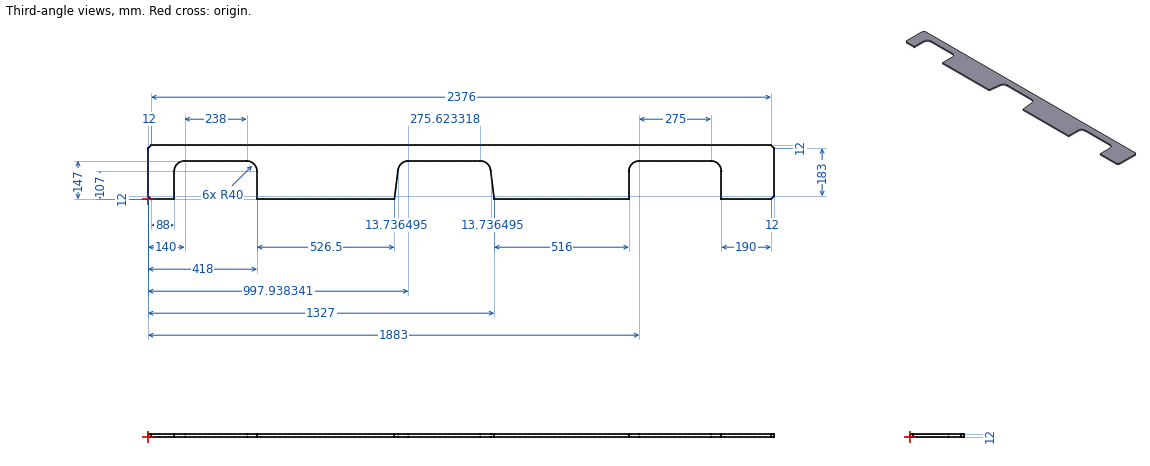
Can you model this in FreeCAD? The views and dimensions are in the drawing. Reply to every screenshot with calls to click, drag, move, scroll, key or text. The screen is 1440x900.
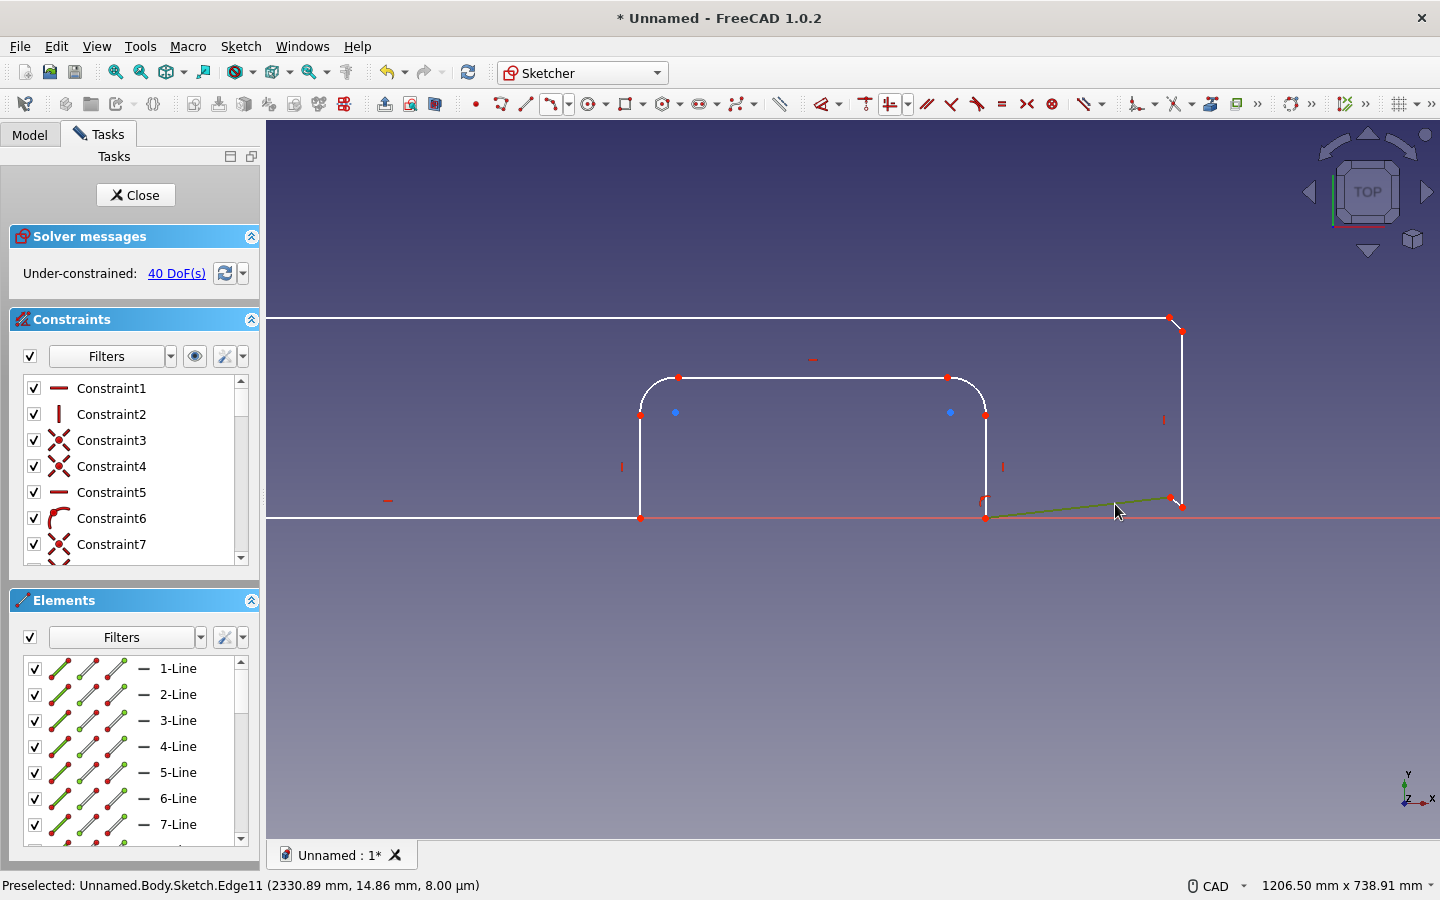
click(908, 104)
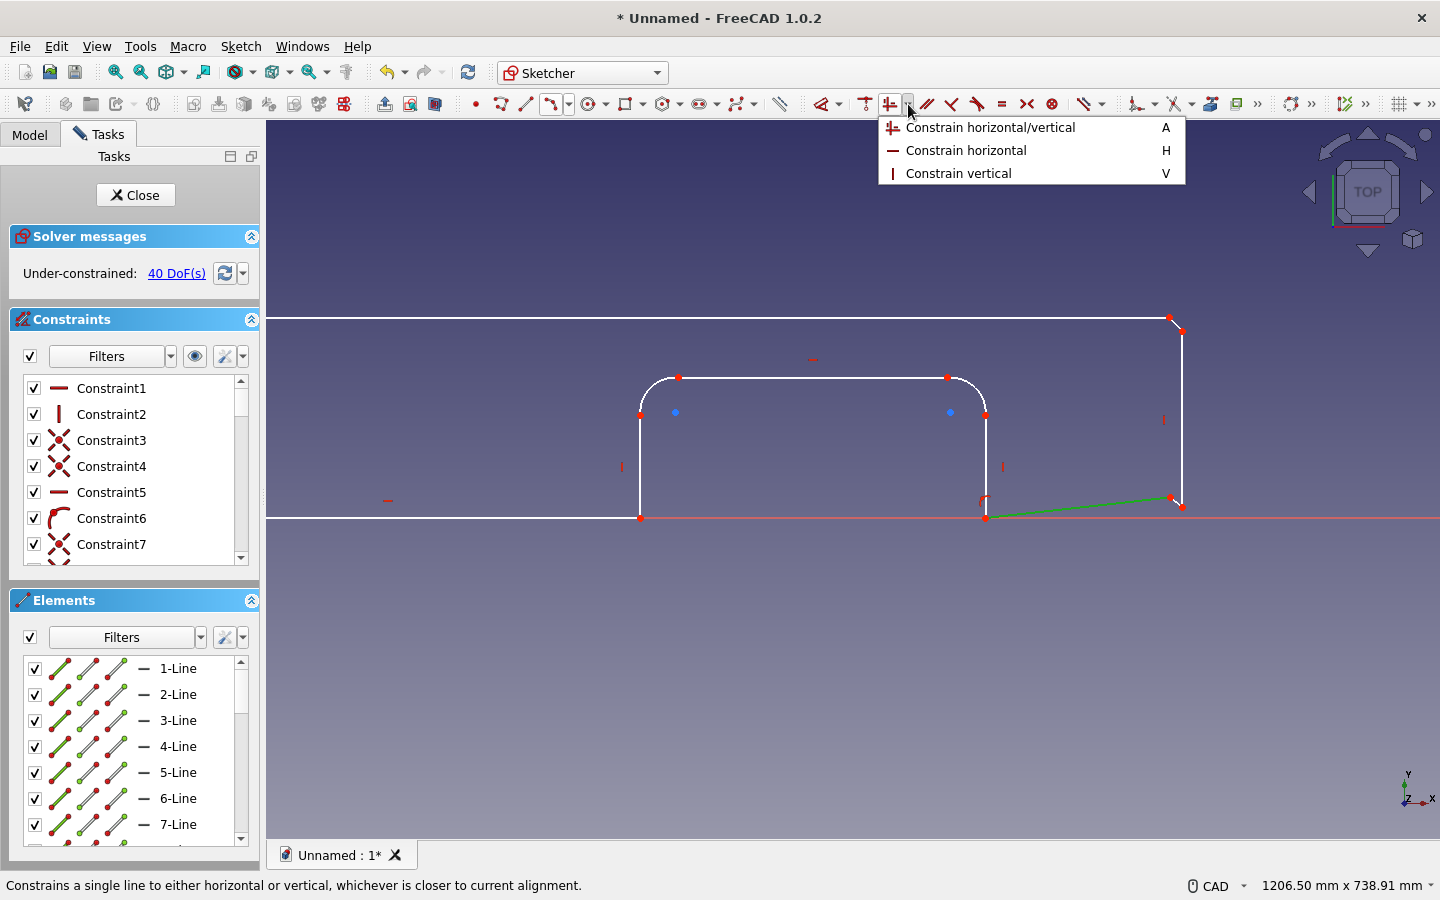
click(1032, 150)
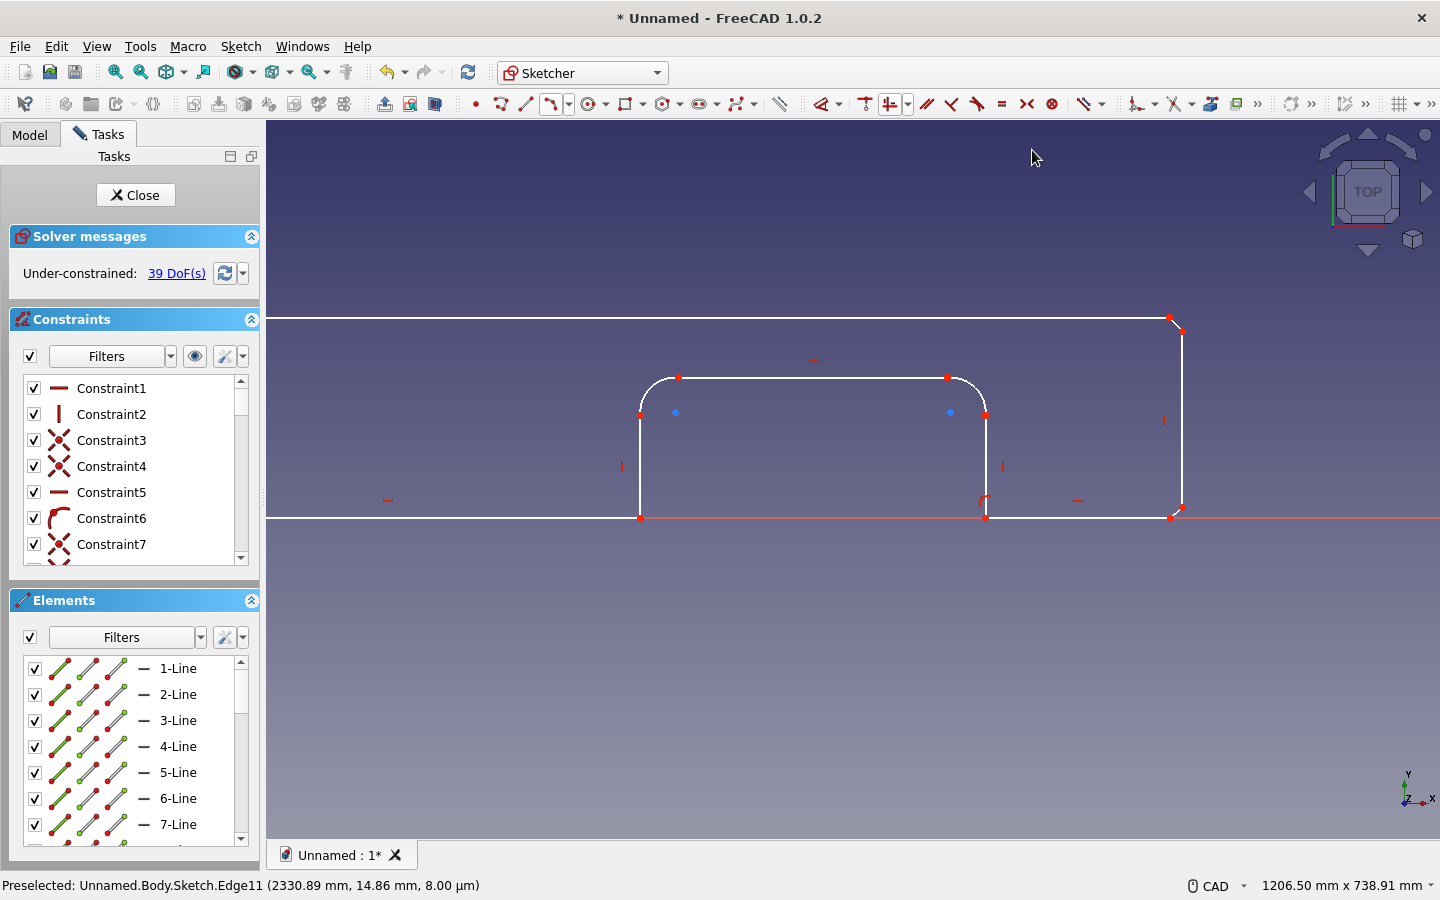
scroll(1116, 506, down, 6)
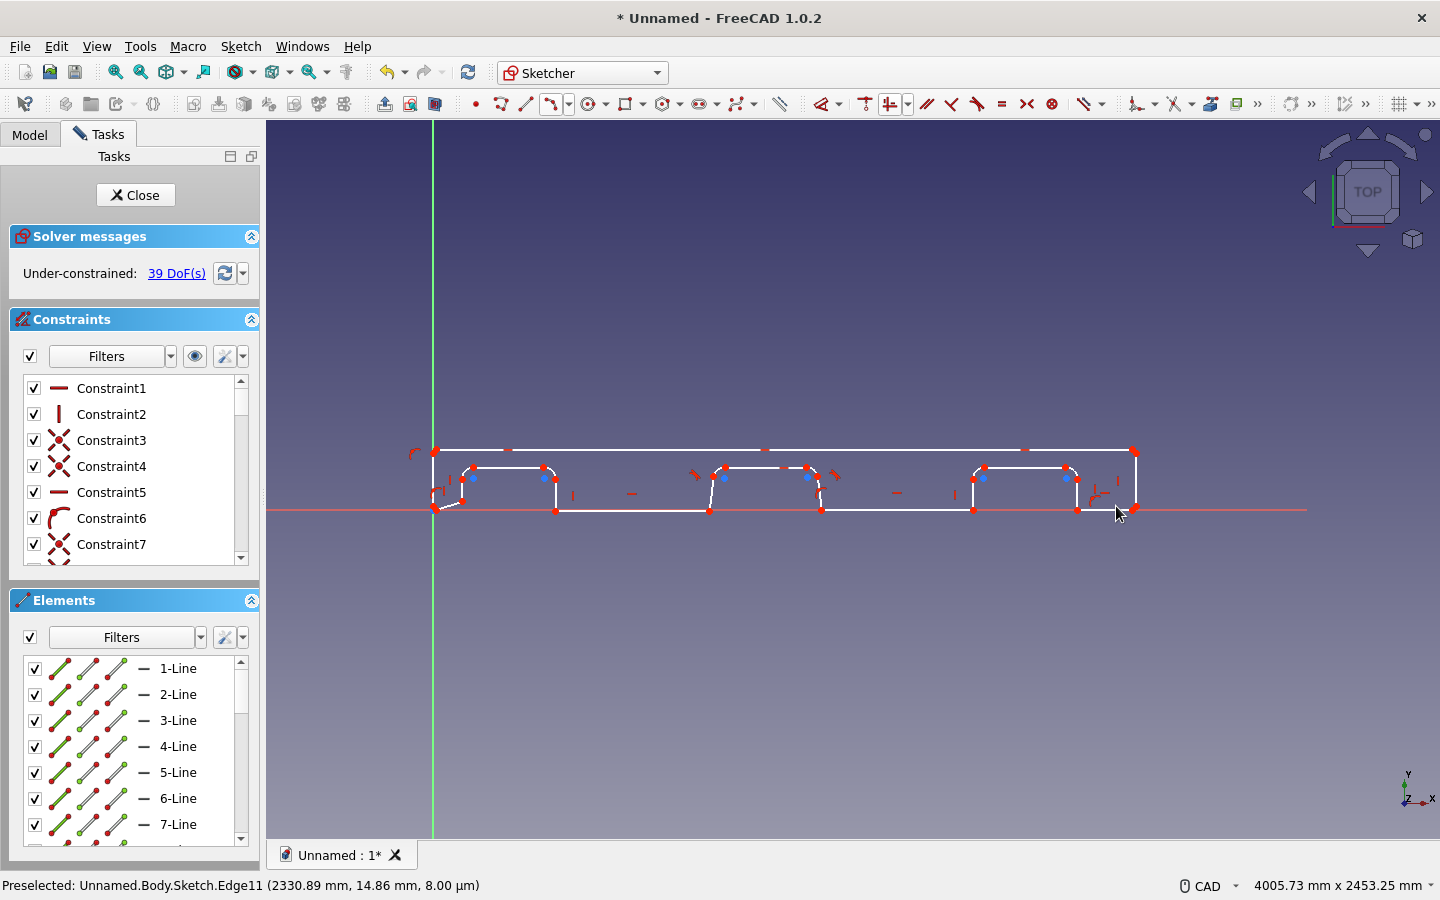
scroll(455, 504, up, 5)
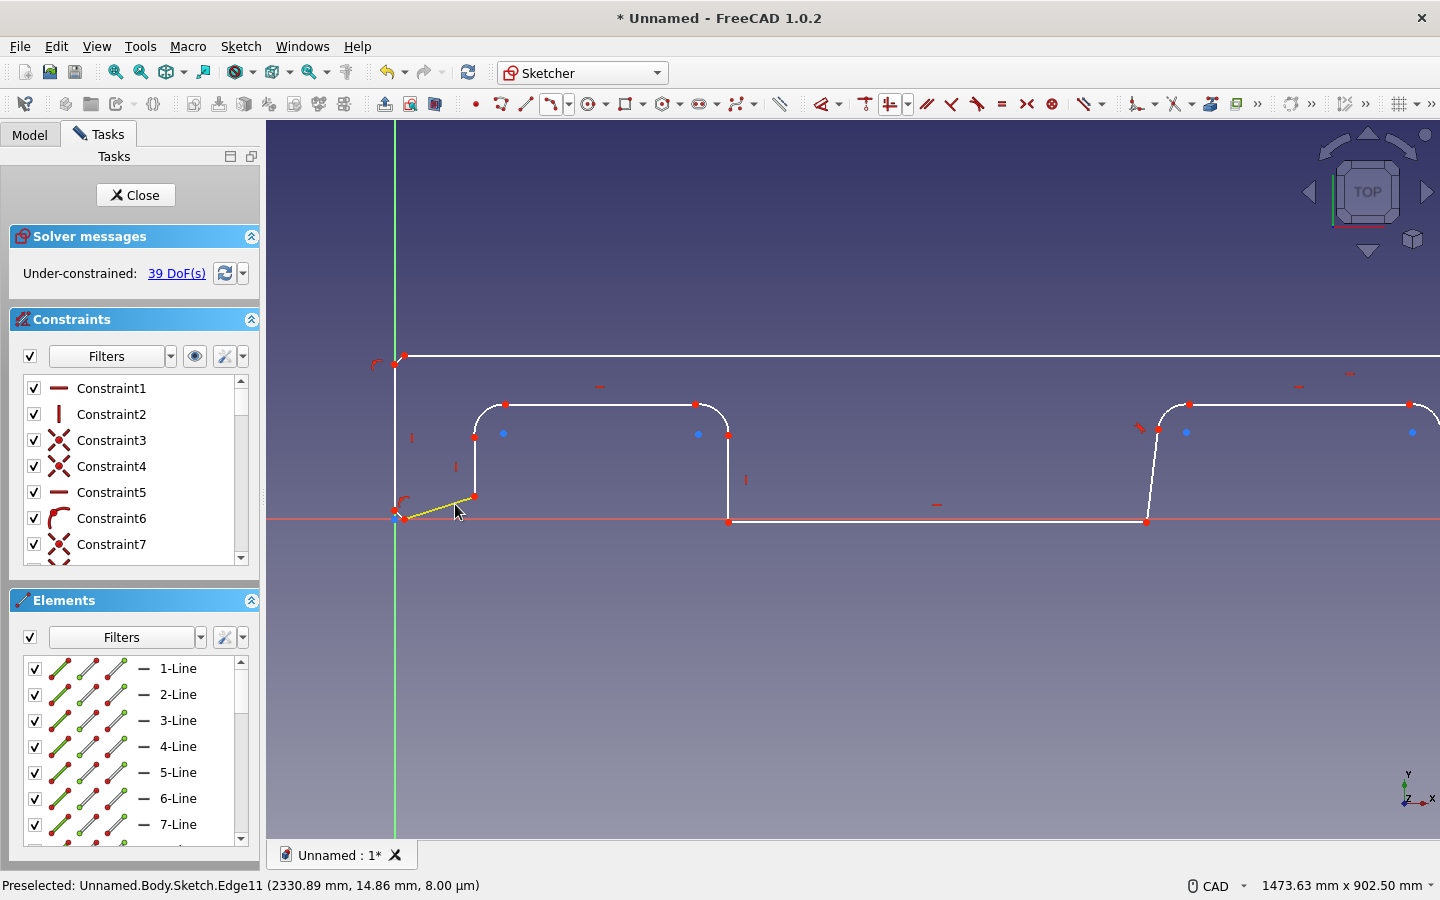
click(454, 504)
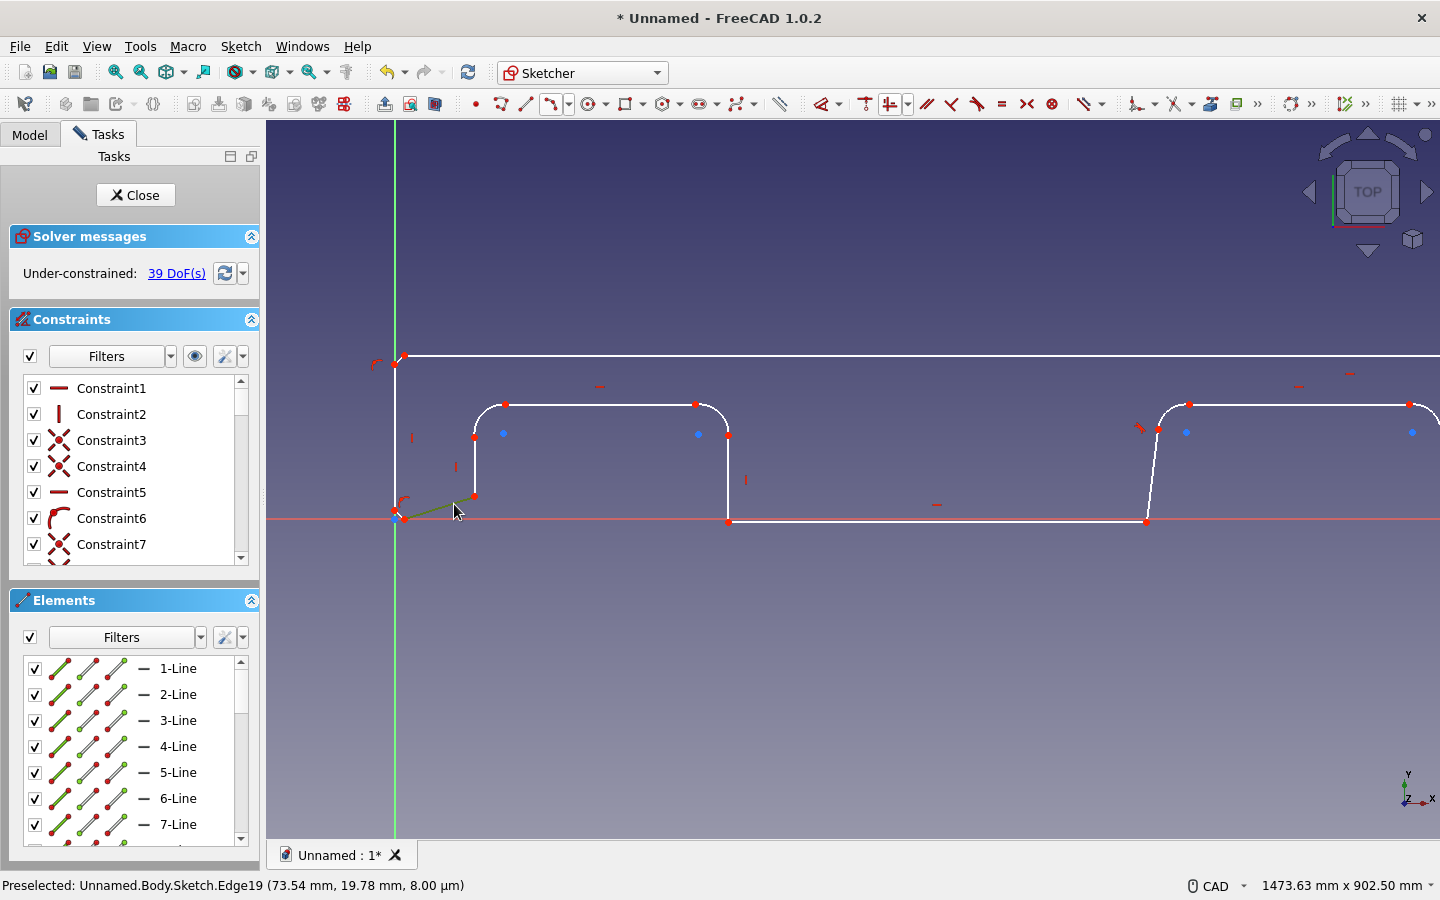
click(908, 104)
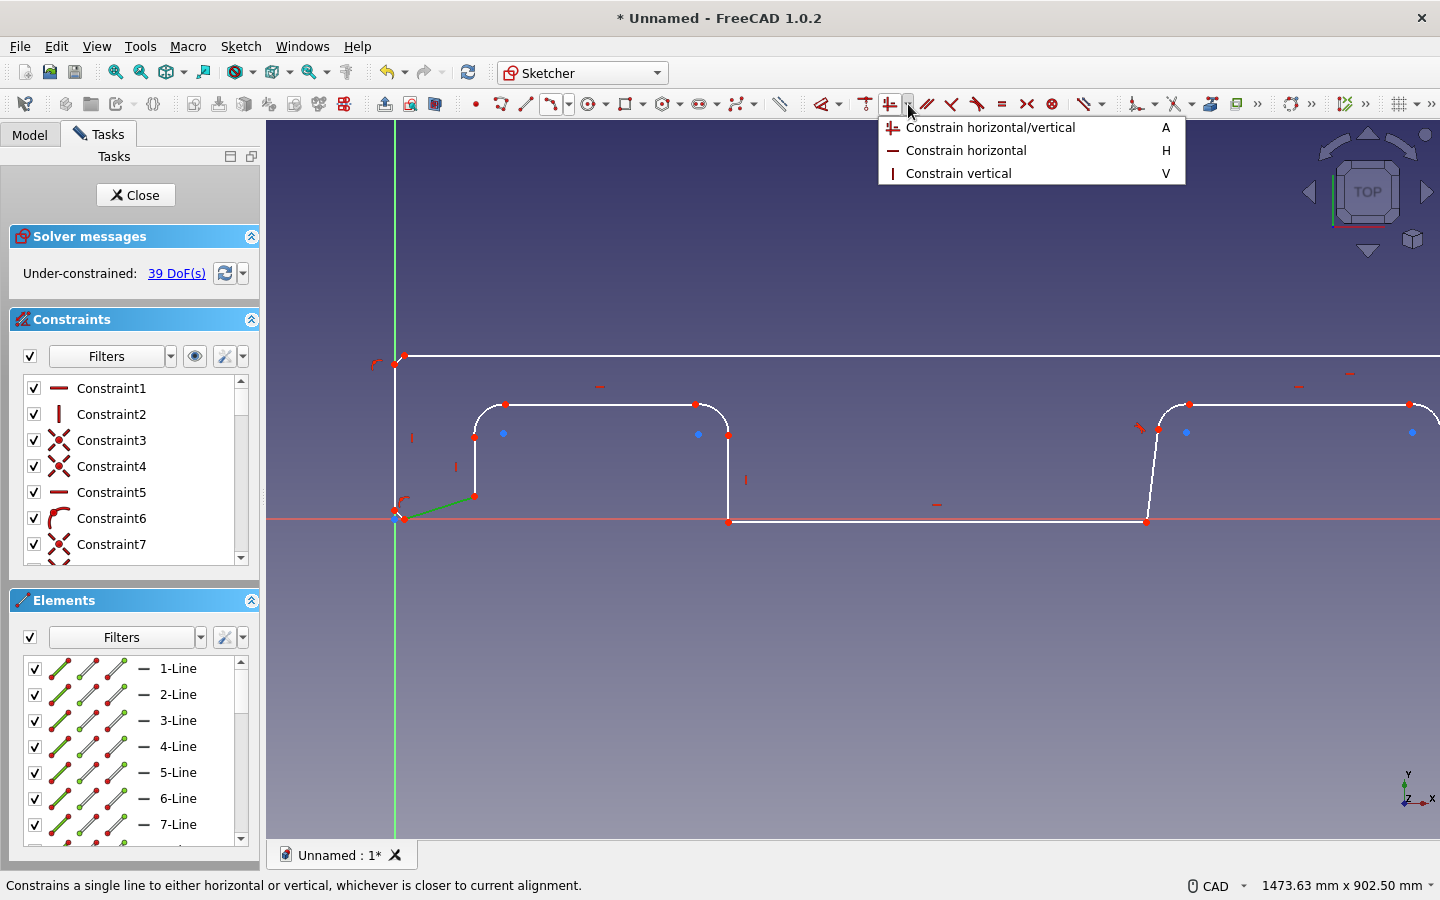
click(1032, 150)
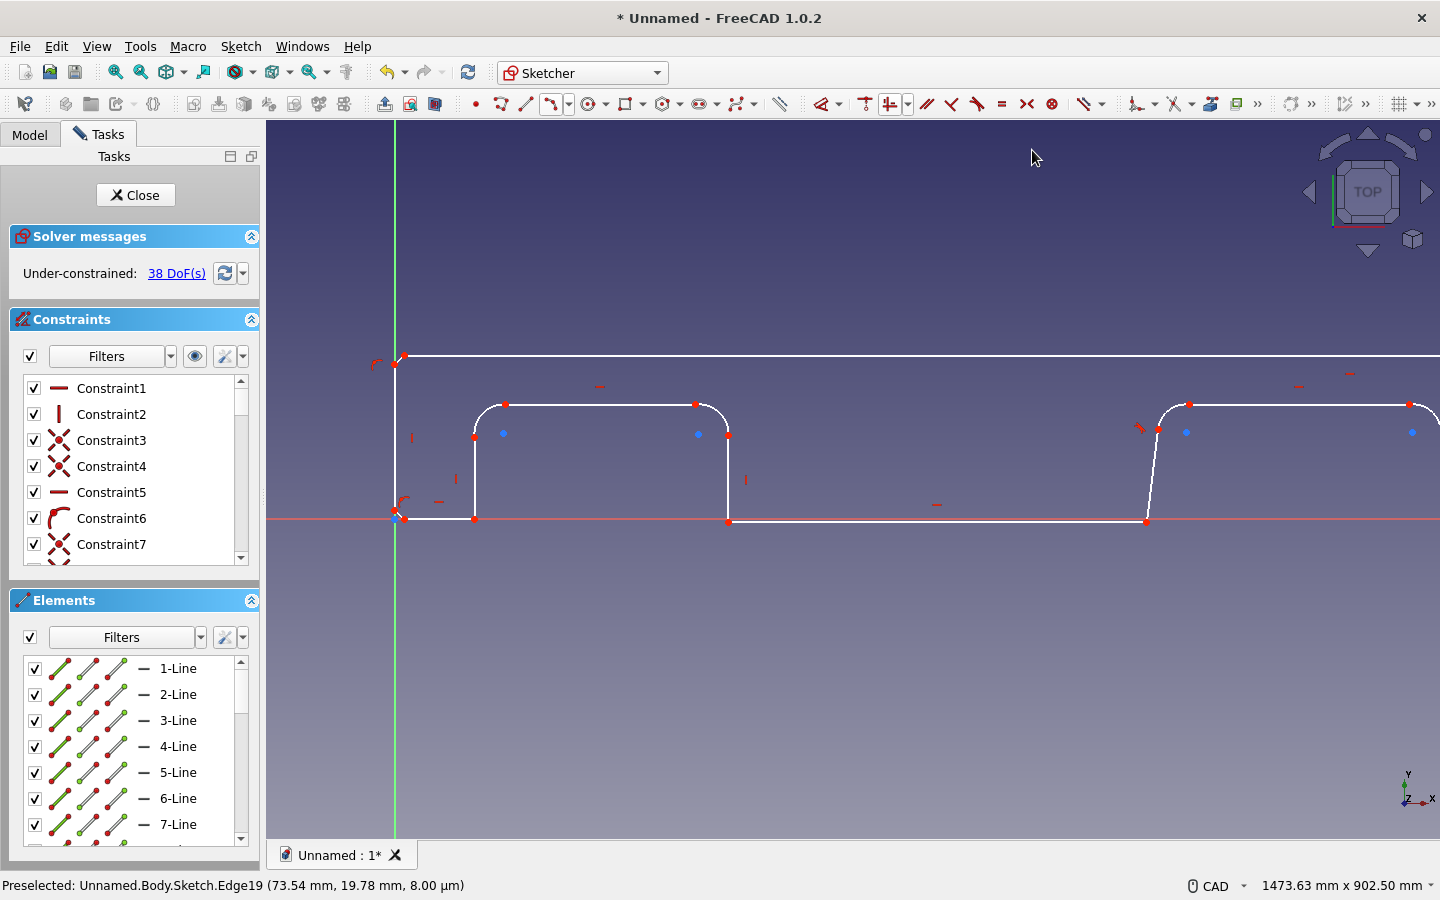
click(725, 421)